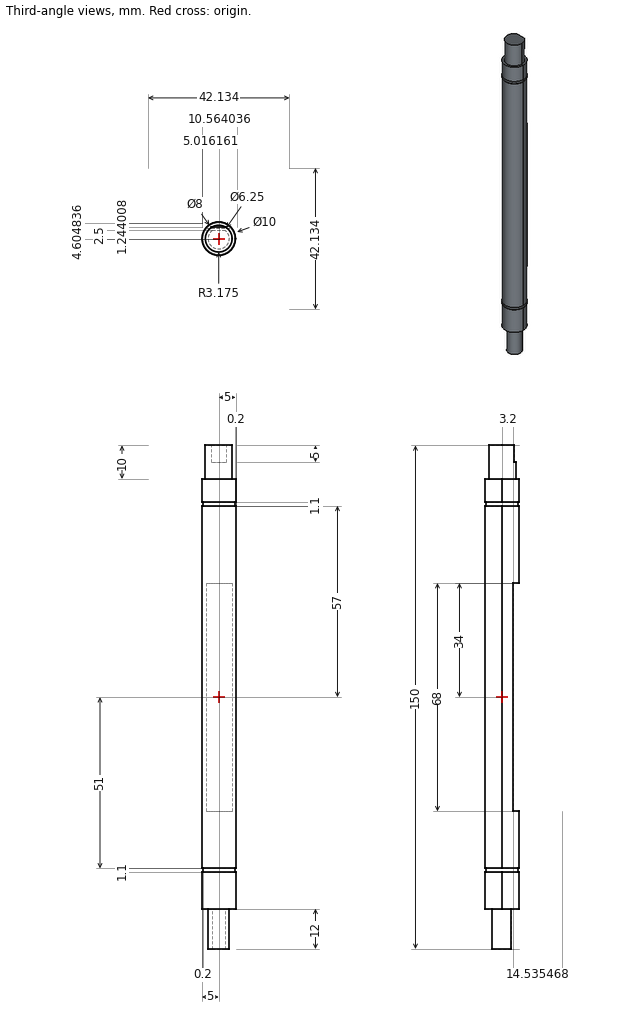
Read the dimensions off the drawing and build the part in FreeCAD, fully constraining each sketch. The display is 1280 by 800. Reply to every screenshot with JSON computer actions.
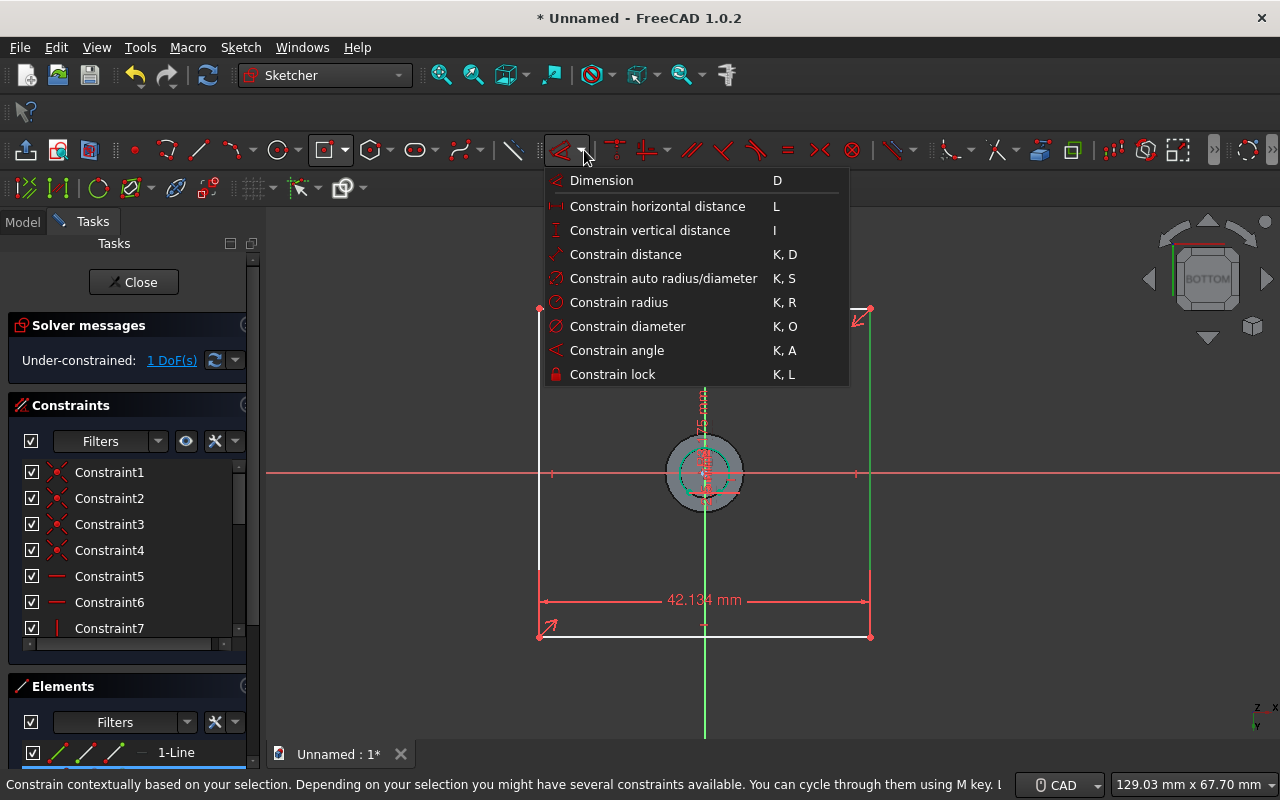
{"action": "left_click", "coordinate": [697, 230]}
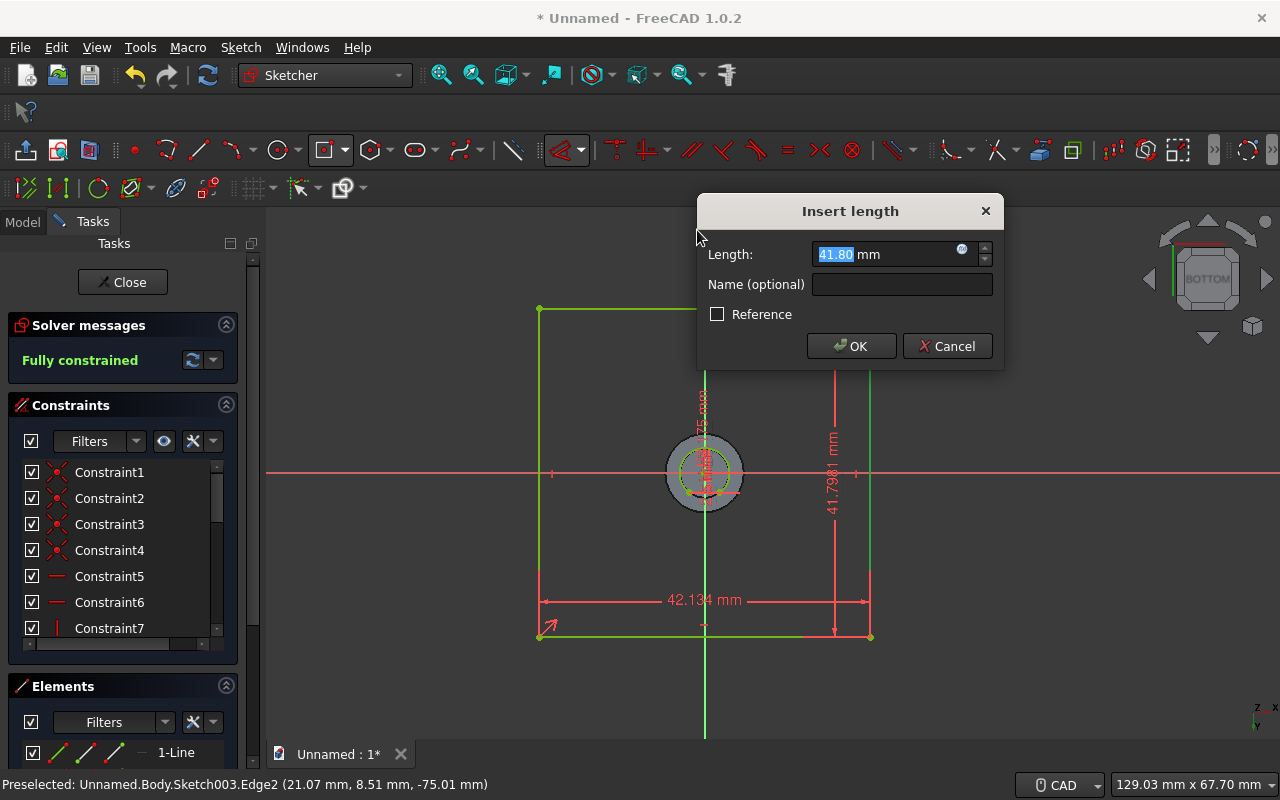
{"action": "type", "text": "42.134"}
{"action": "key", "text": "Return"}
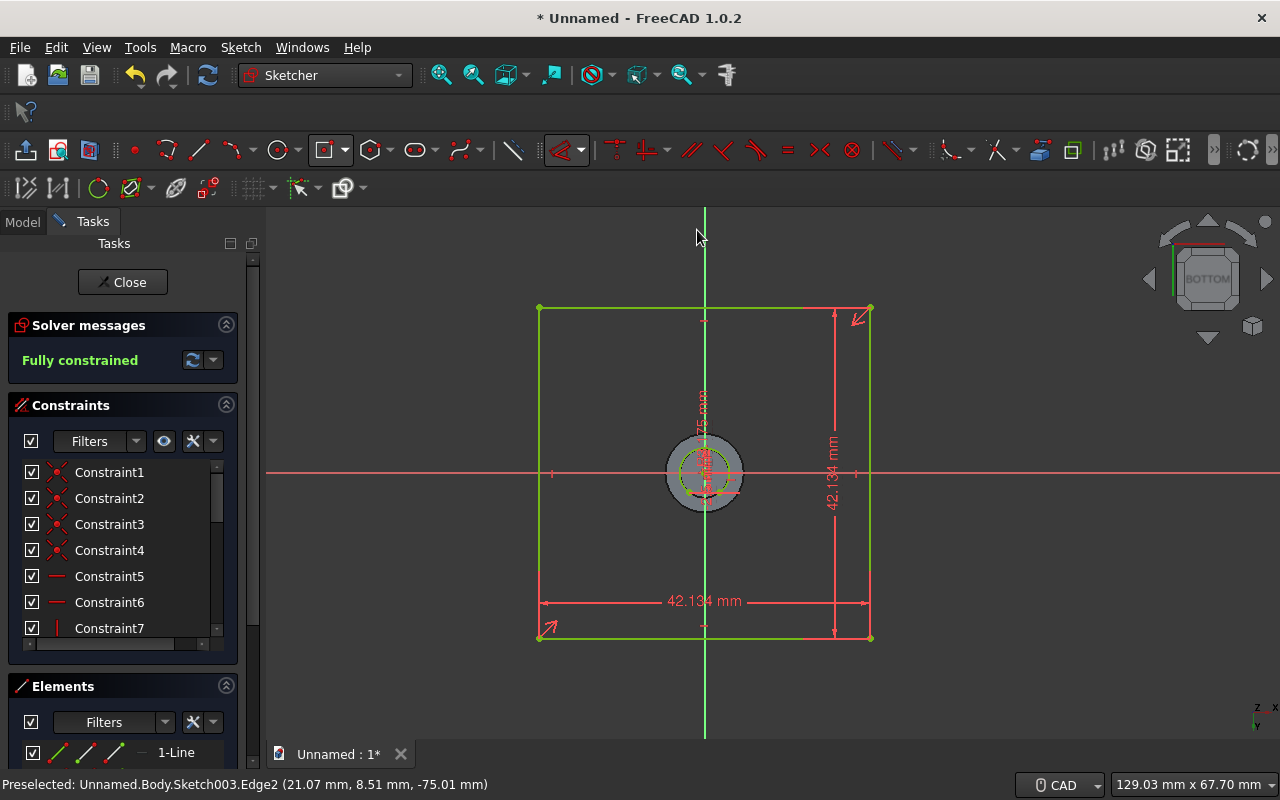
{"action": "left_click", "coordinate": [123, 282]}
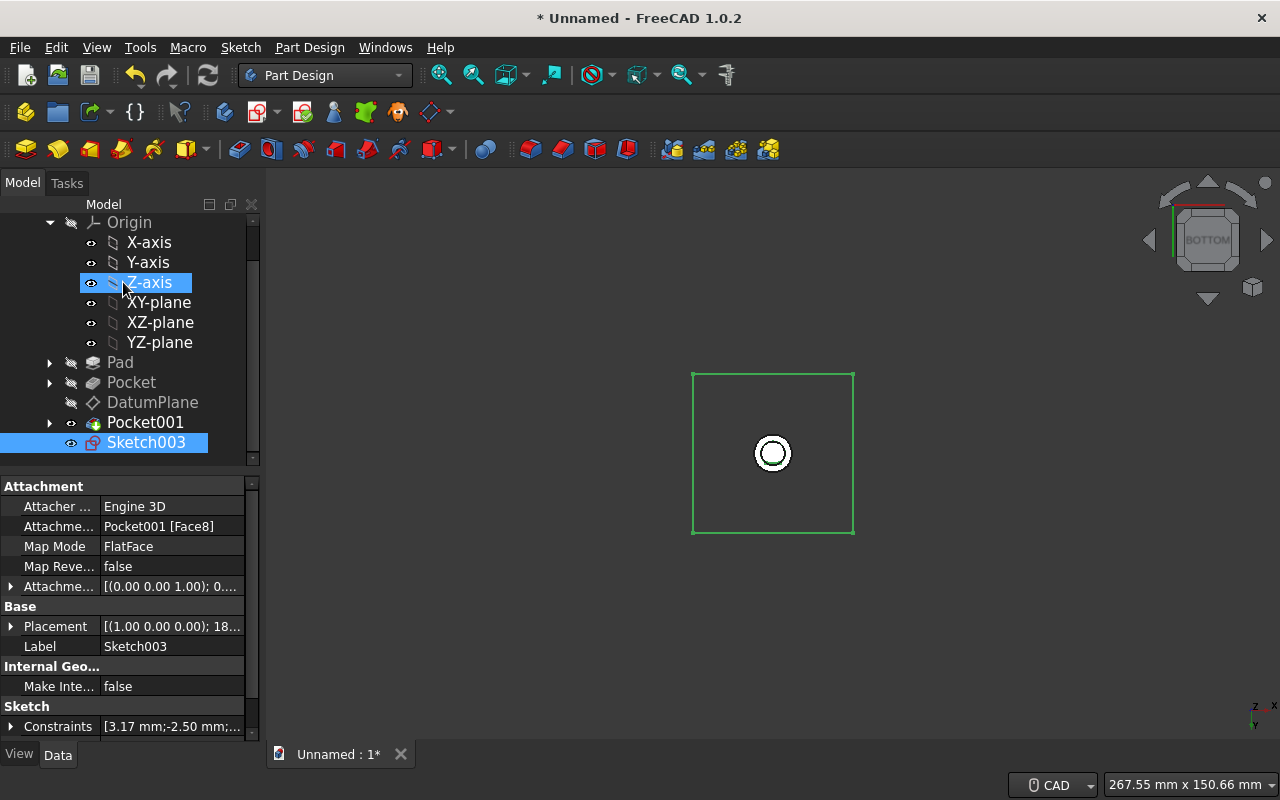
{"action": "left_click", "coordinate": [240, 150]}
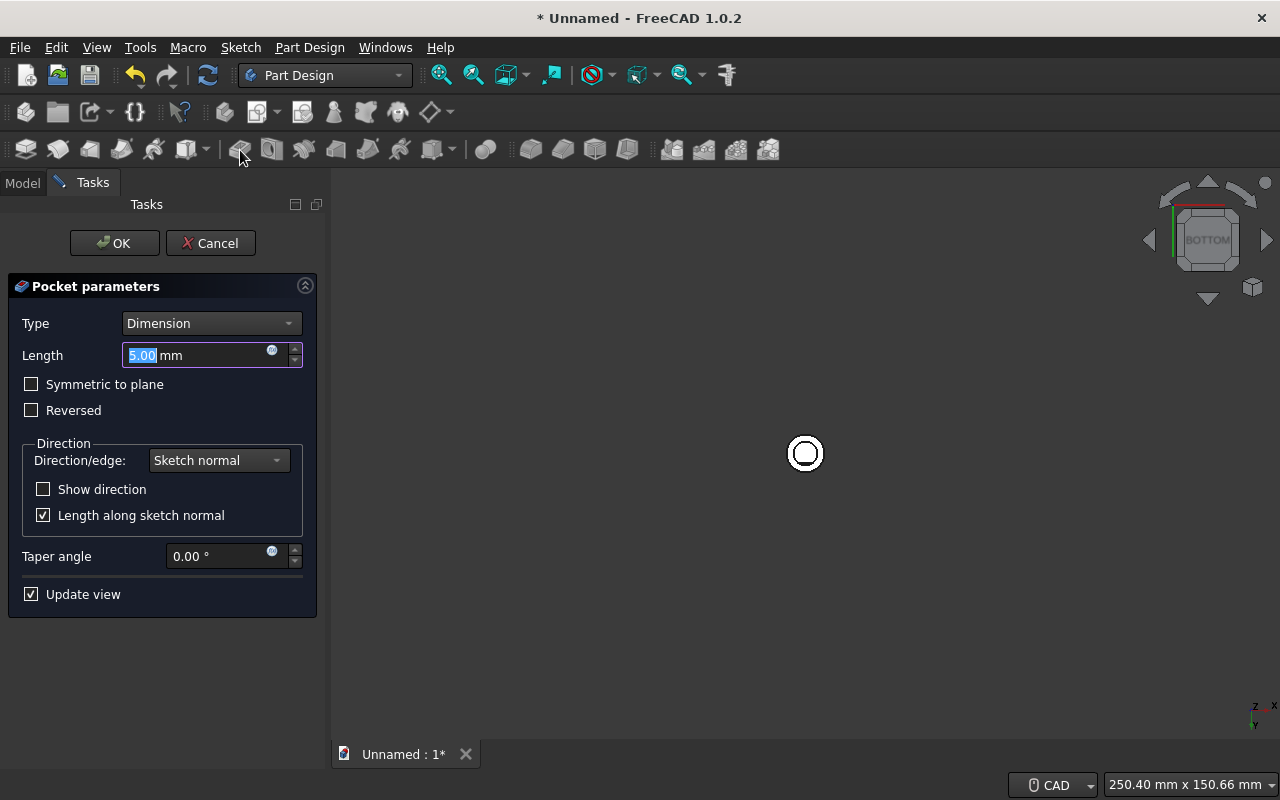
{"action": "type", "text": "12"}
{"action": "key", "text": "Tab"}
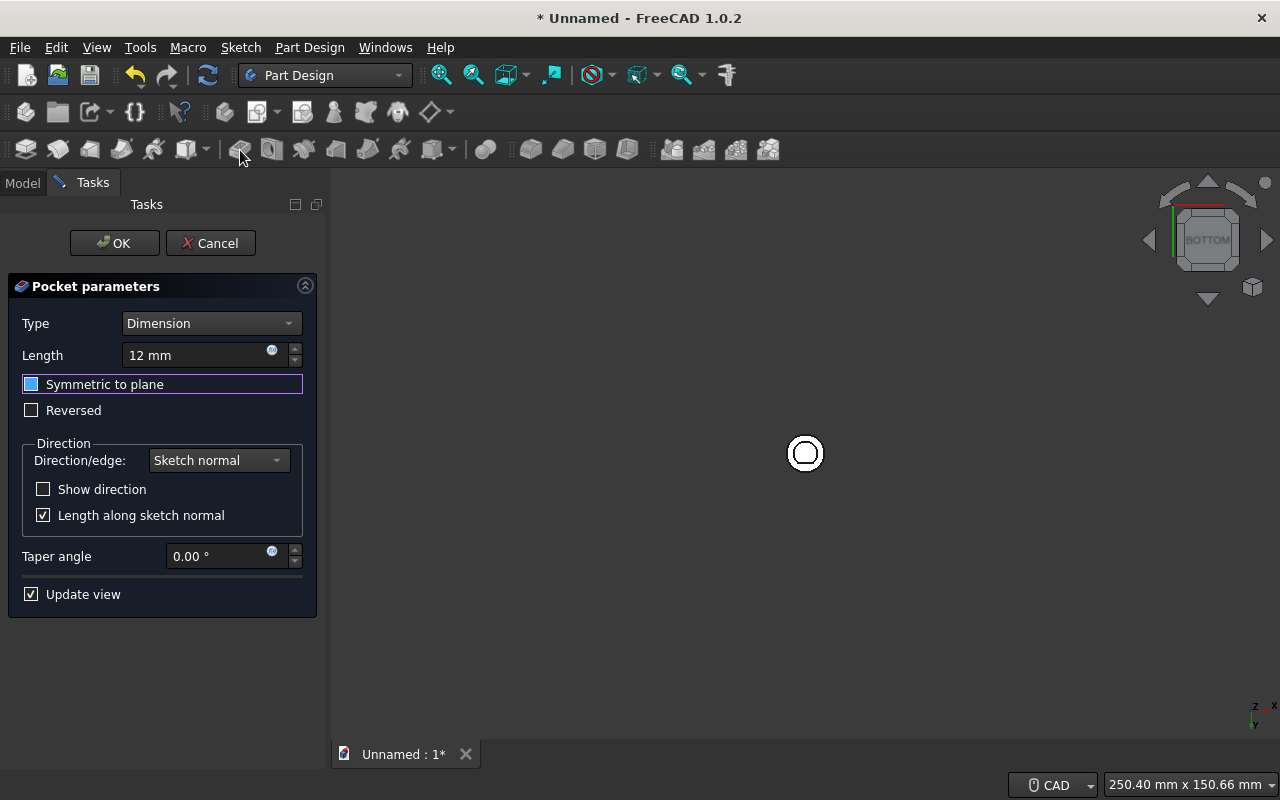
{"action": "left_click", "coordinate": [115, 243]}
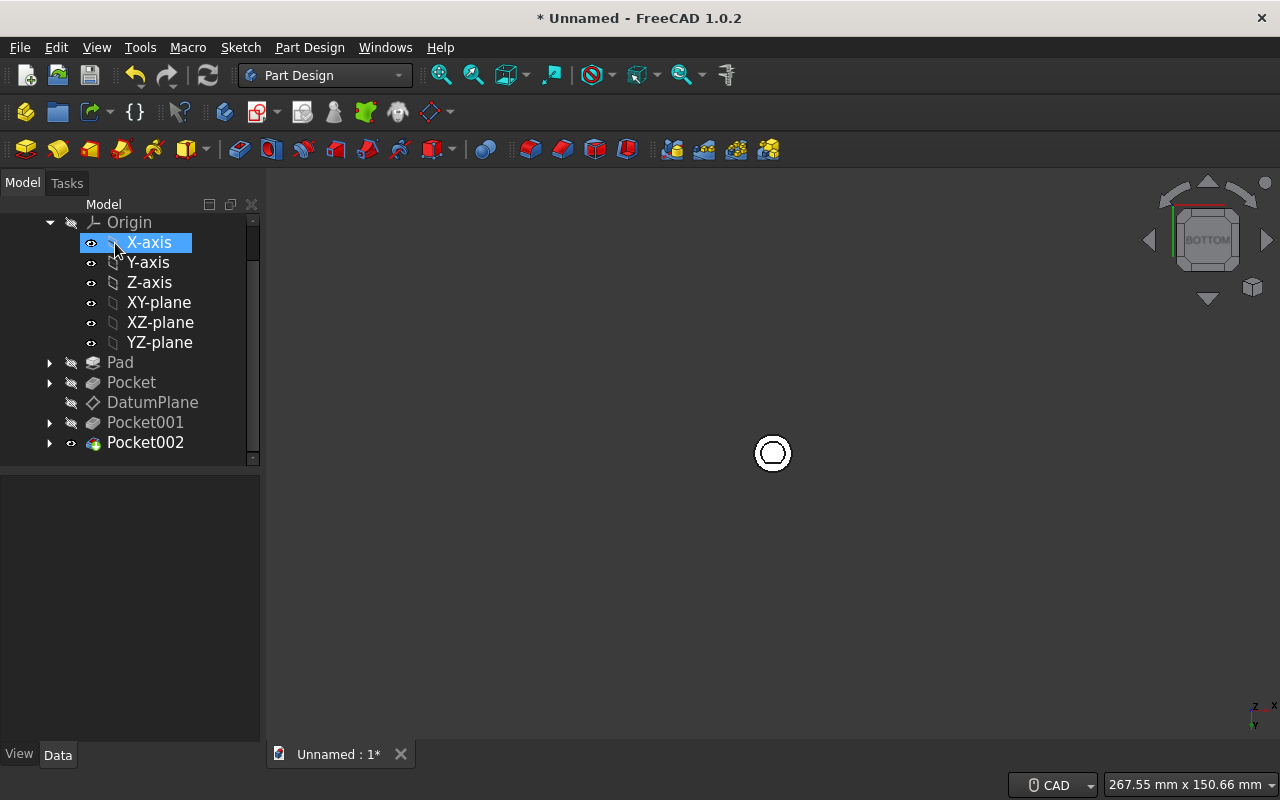
{"action": "left_click", "coordinate": [442, 76]}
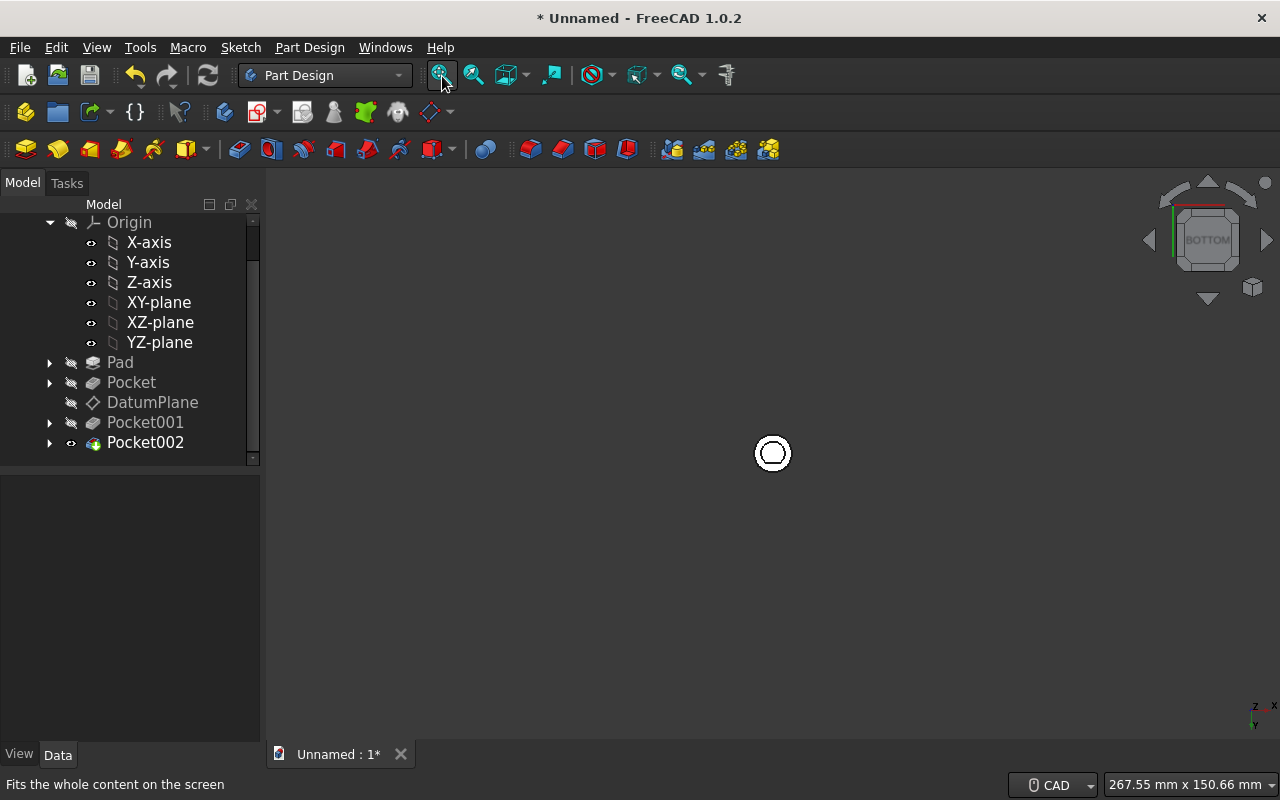
{"action": "key", "text": "0"}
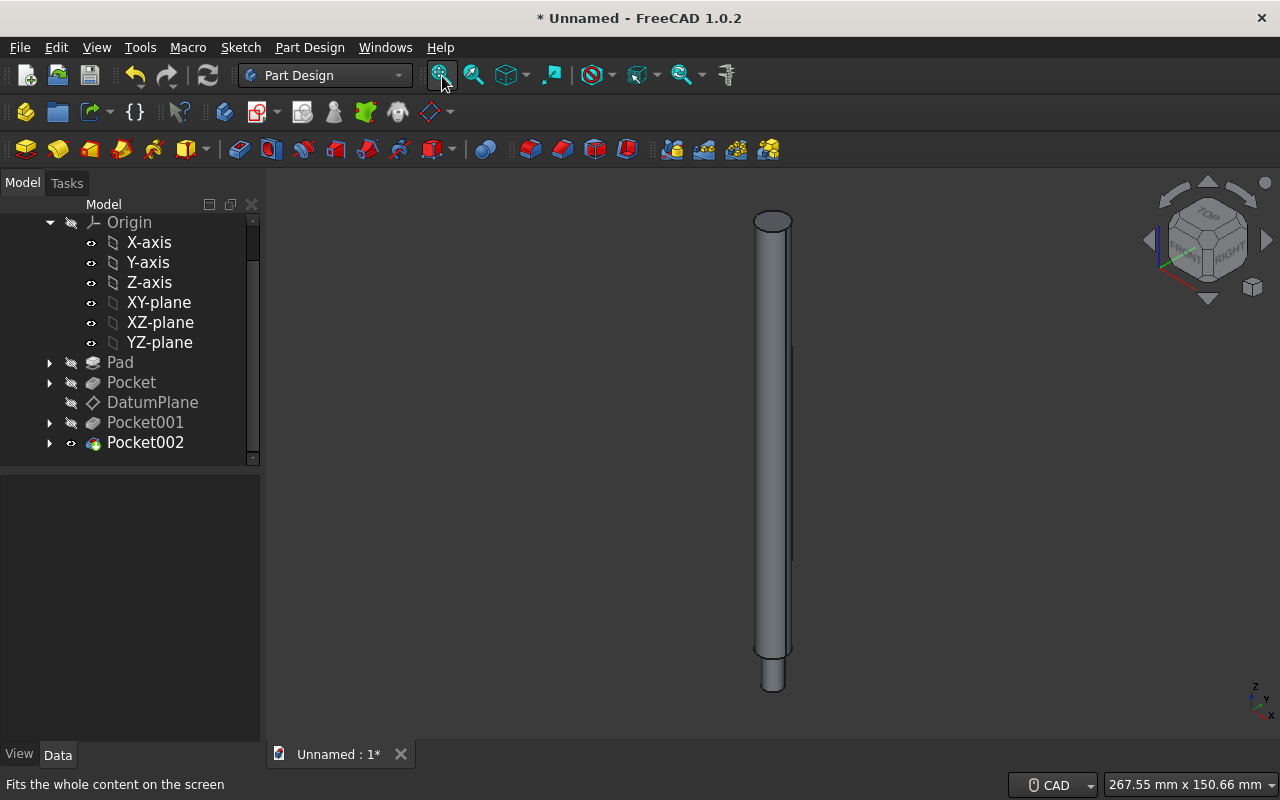
{"action": "left_click", "coordinate": [773, 220]}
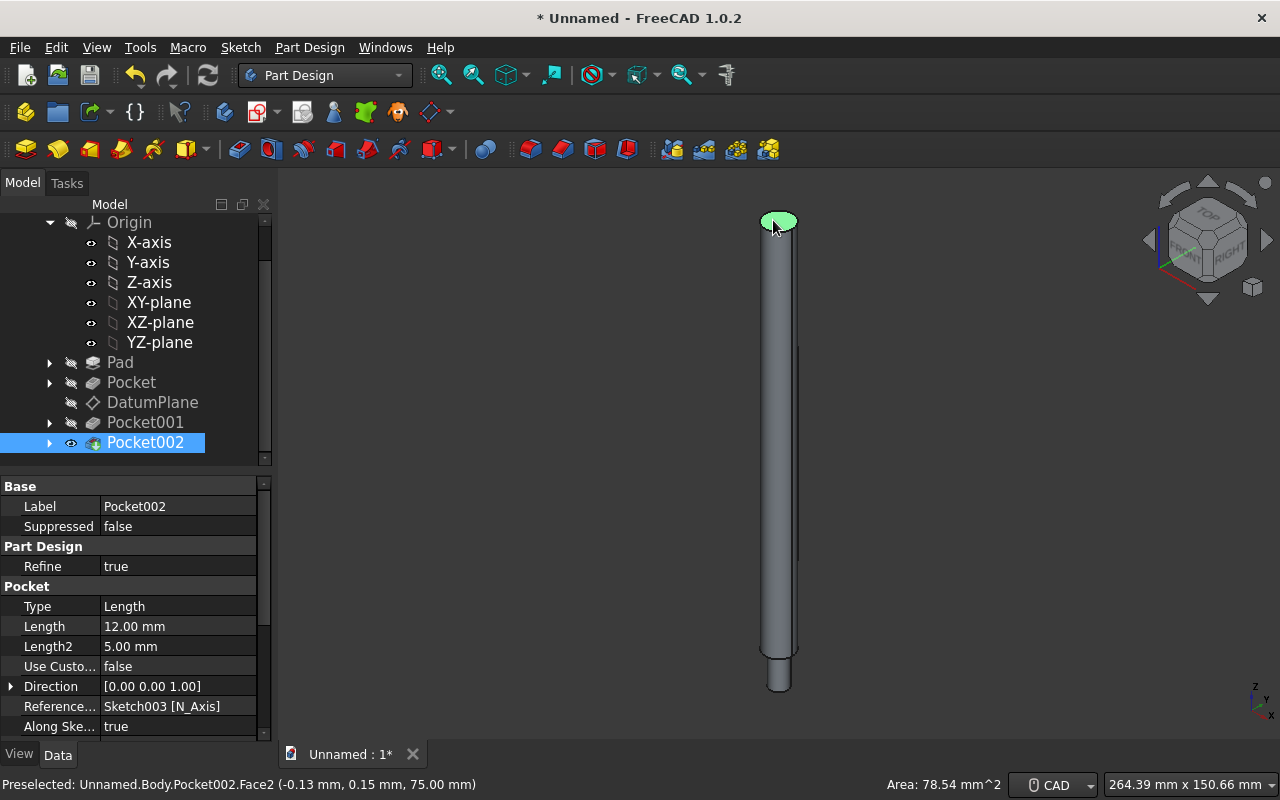
{"action": "left_click", "coordinate": [258, 112]}